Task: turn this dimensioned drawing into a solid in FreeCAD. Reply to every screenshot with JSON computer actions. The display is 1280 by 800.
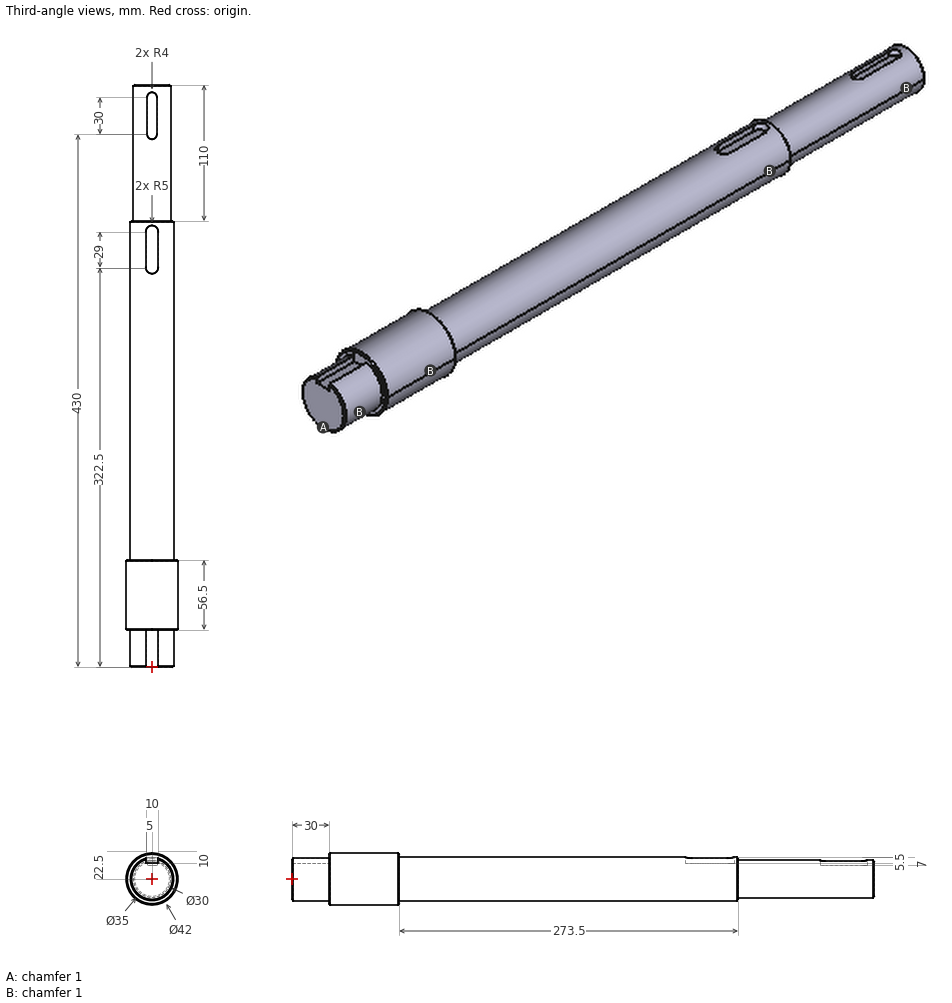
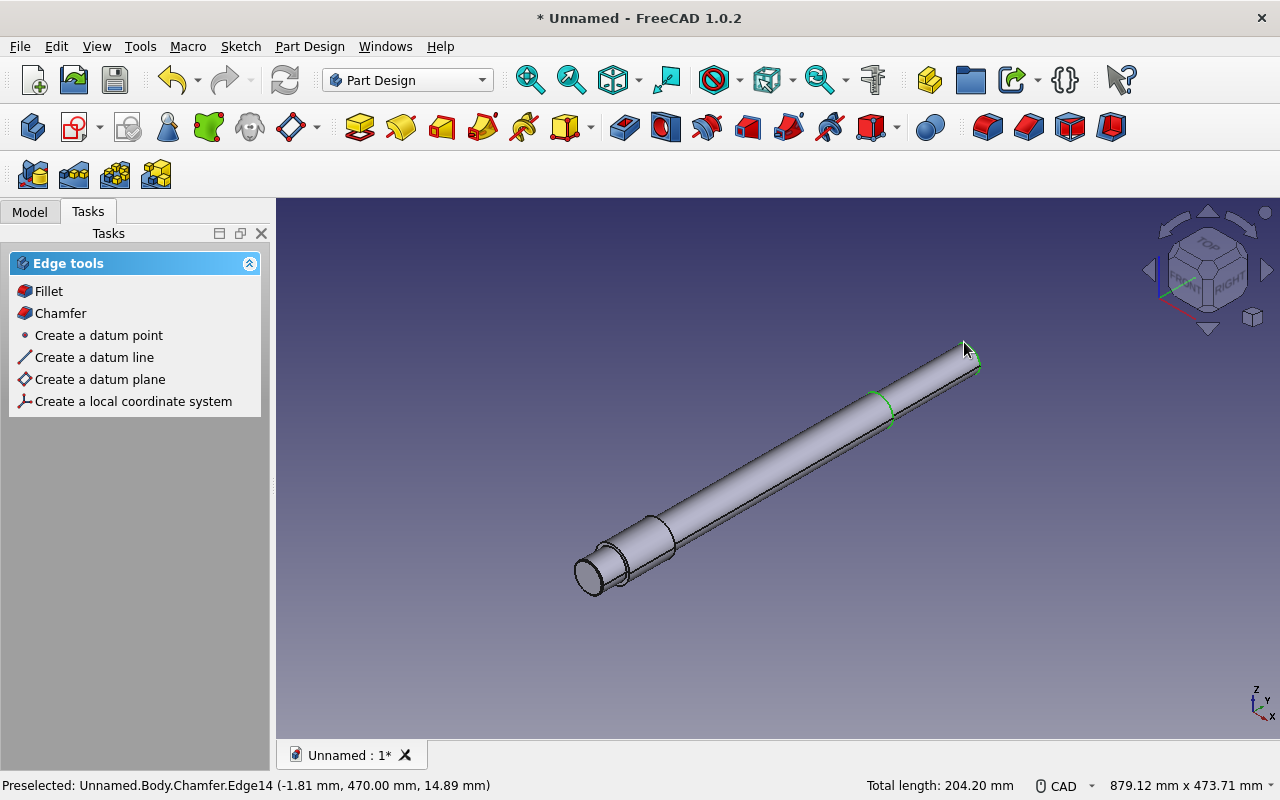
{"action": "left_click", "coordinate": [607, 541], "text": "ctrl"}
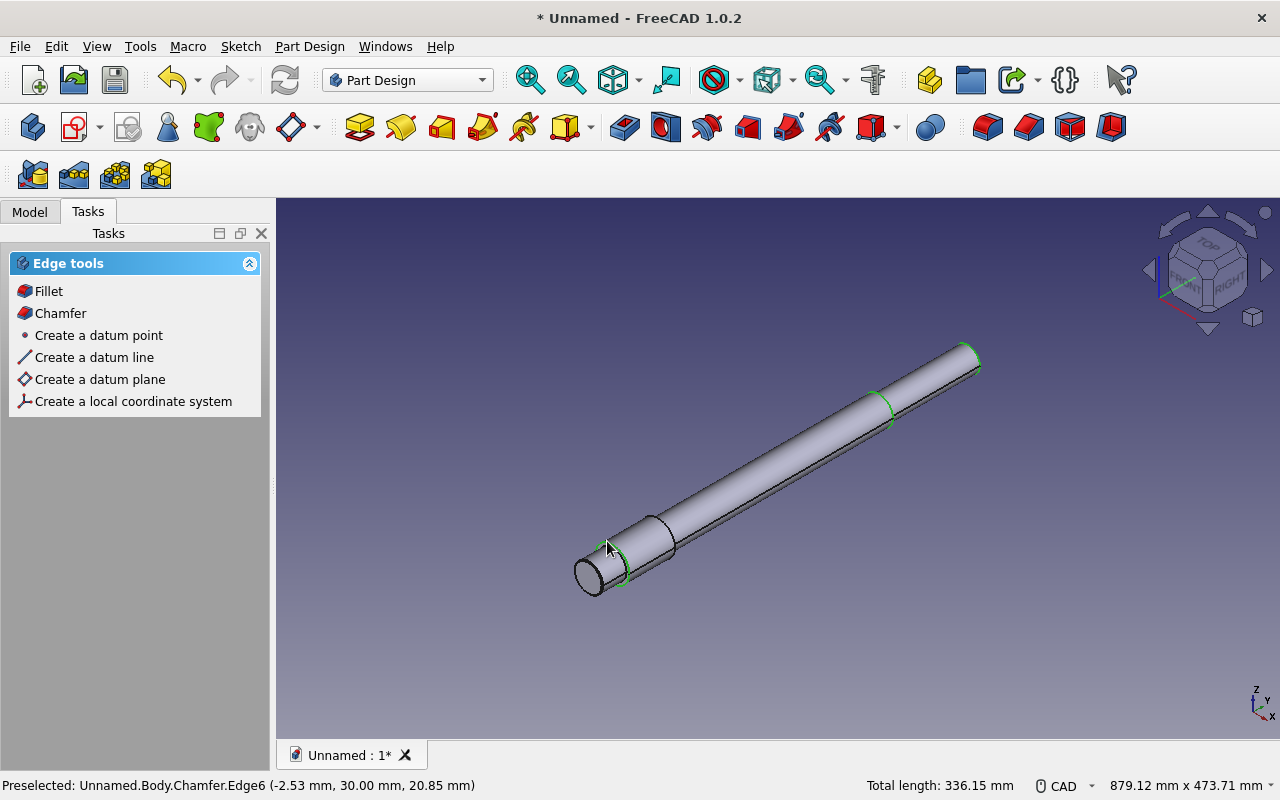
{"action": "left_click", "coordinate": [653, 515], "text": "ctrl"}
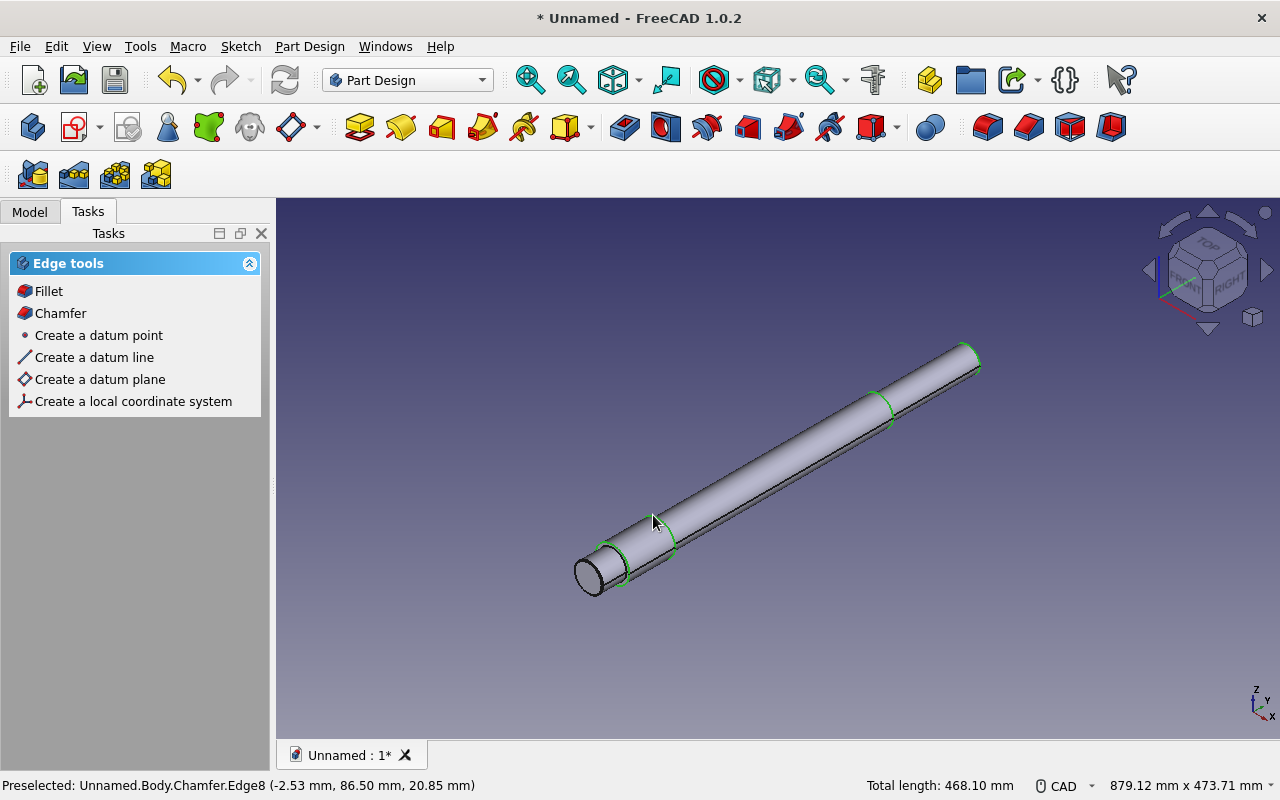
{"action": "left_click", "coordinate": [1029, 128]}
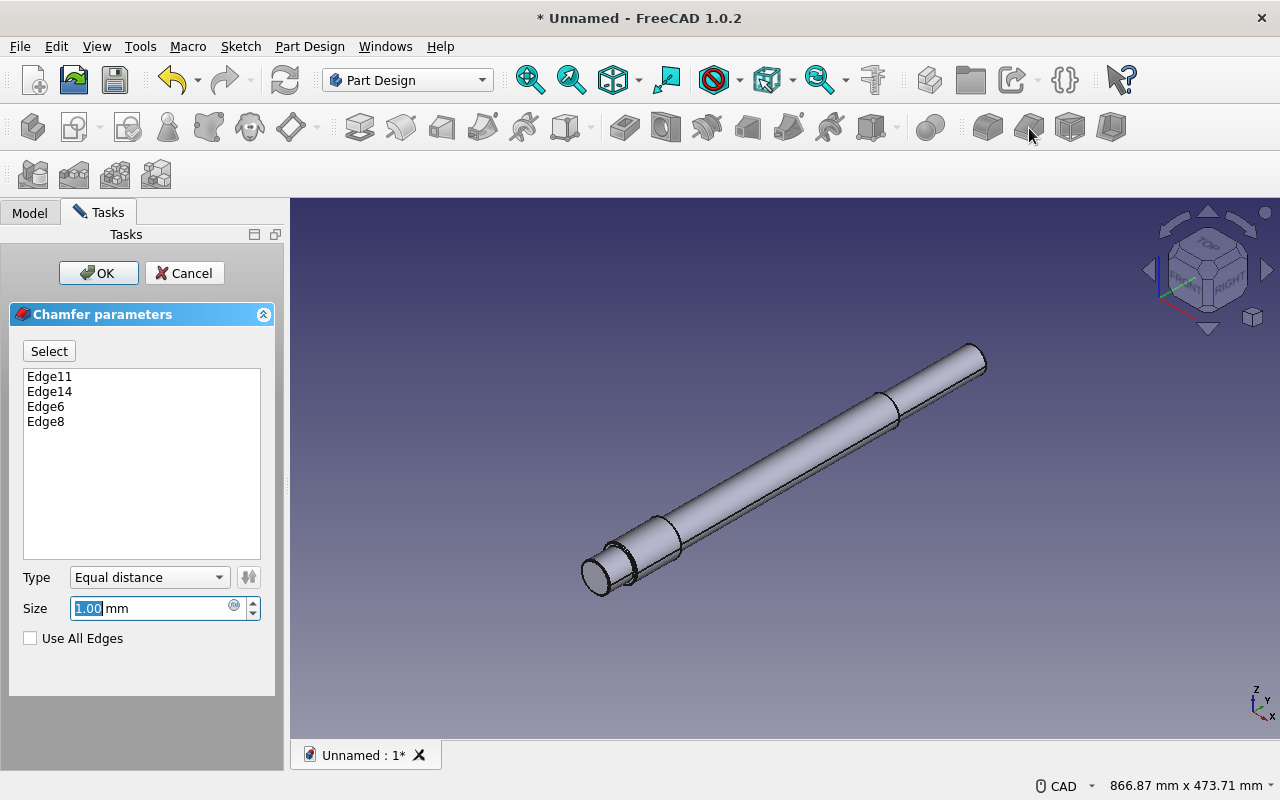
{"action": "type", "text": "1"}
{"action": "key", "text": "Tab"}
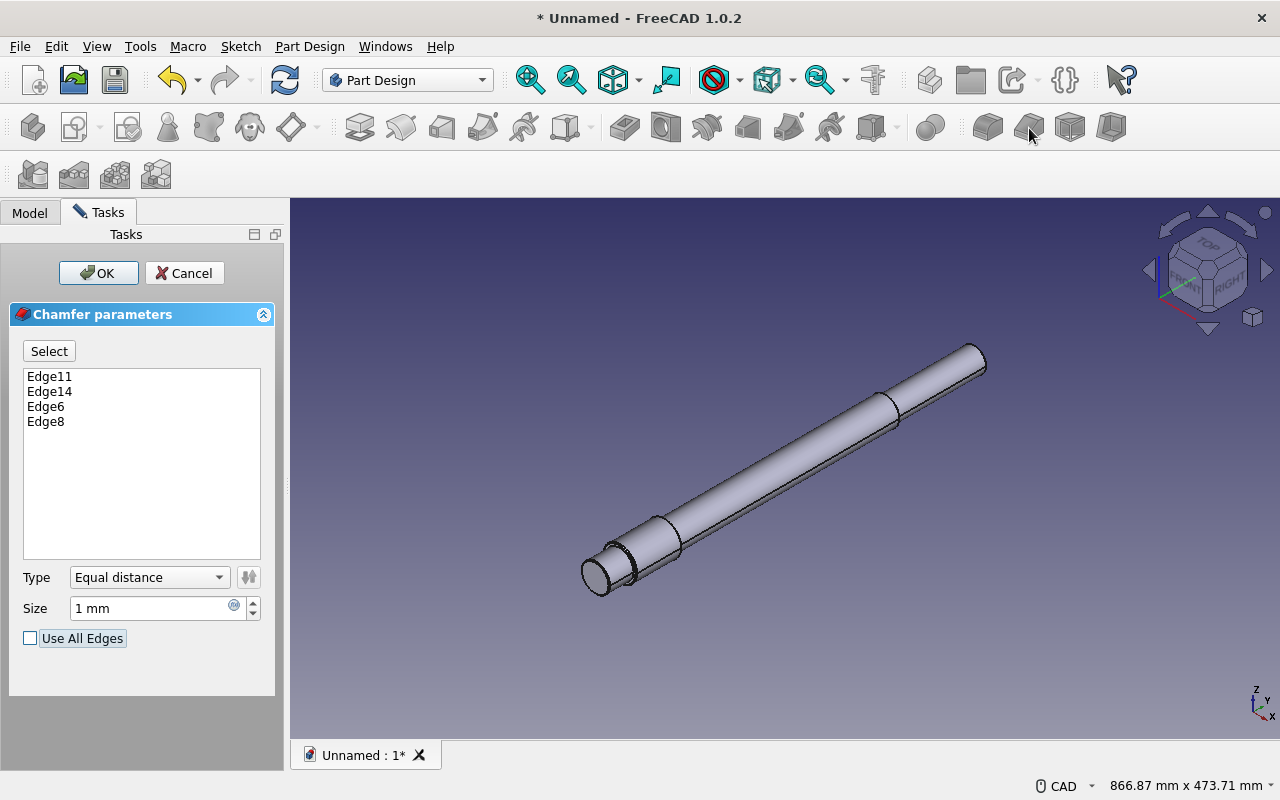
{"action": "left_click", "coordinate": [99, 273]}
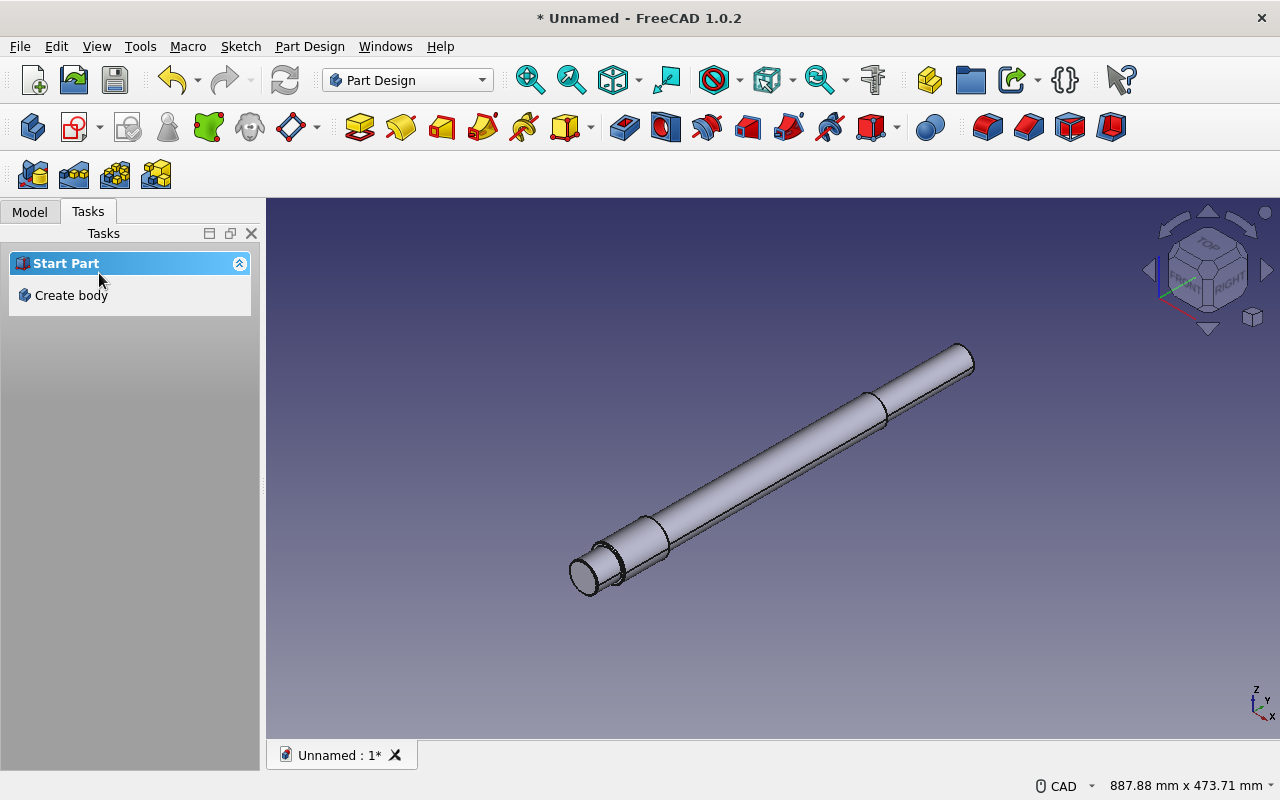
{"action": "left_click", "coordinate": [583, 577]}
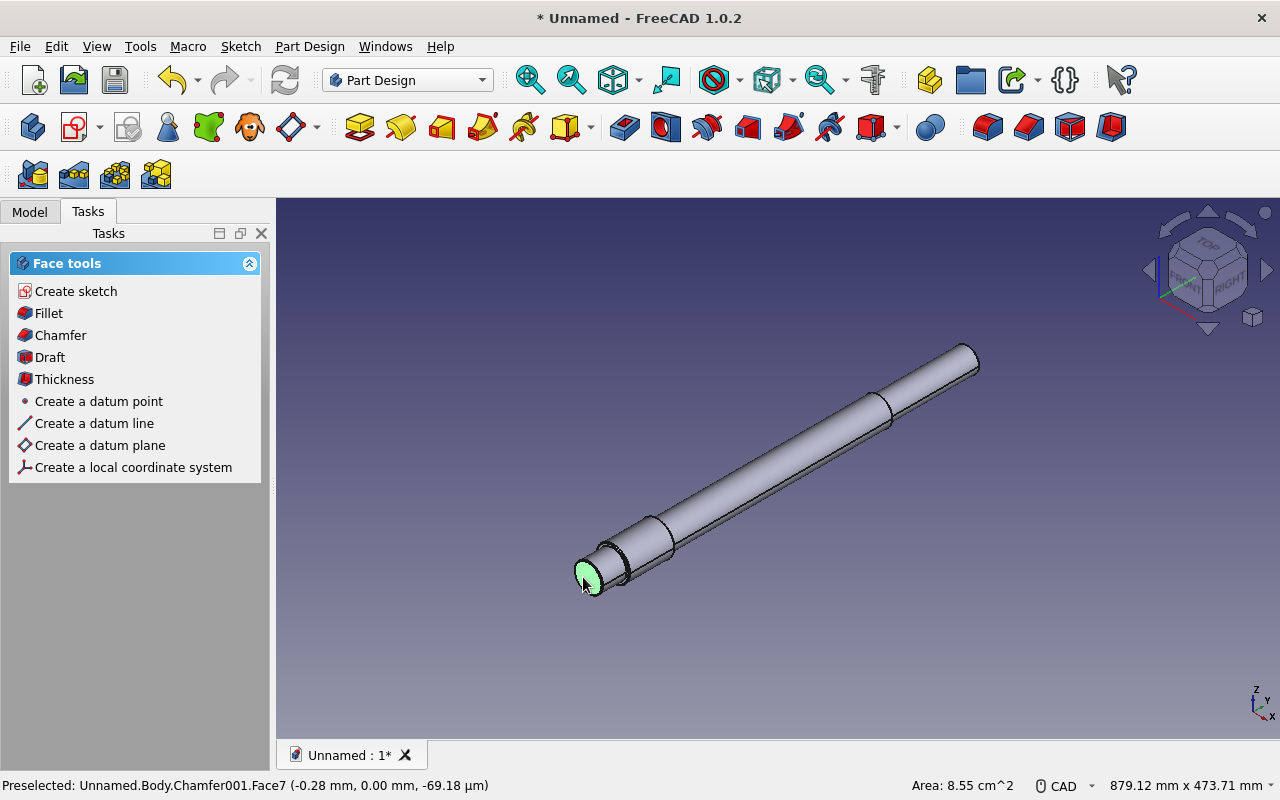
{"action": "left_click", "coordinate": [74, 128]}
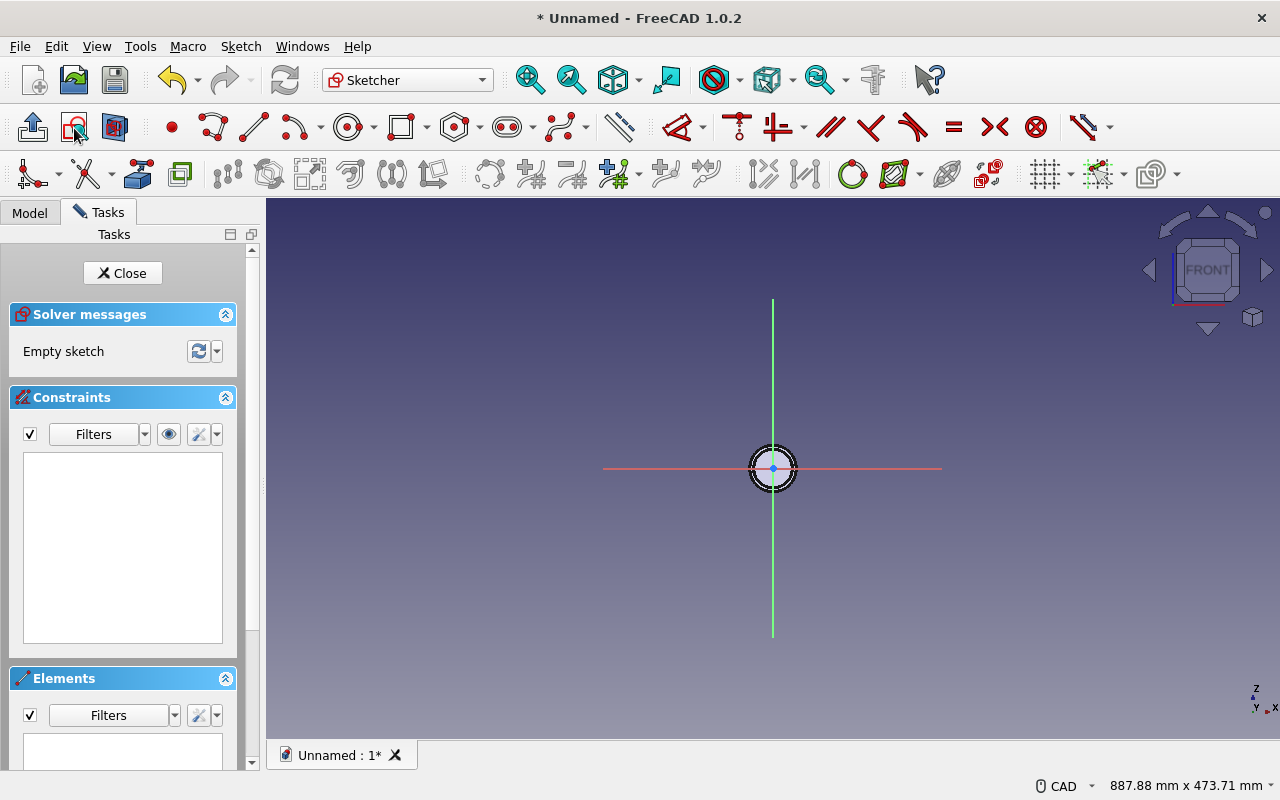
{"action": "scroll", "coordinate": [778, 455], "scroll_direction": "up", "scroll_amount": 13}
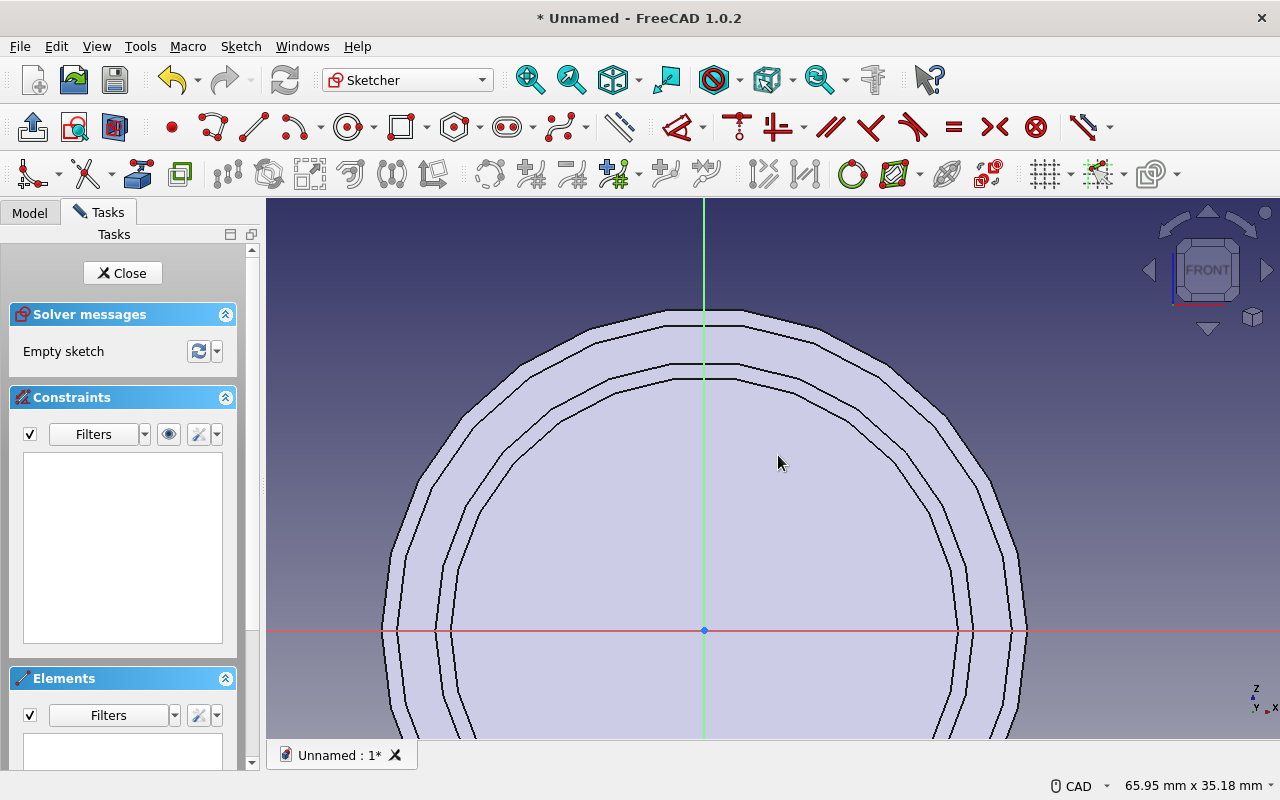
{"action": "key", "text": "g r"}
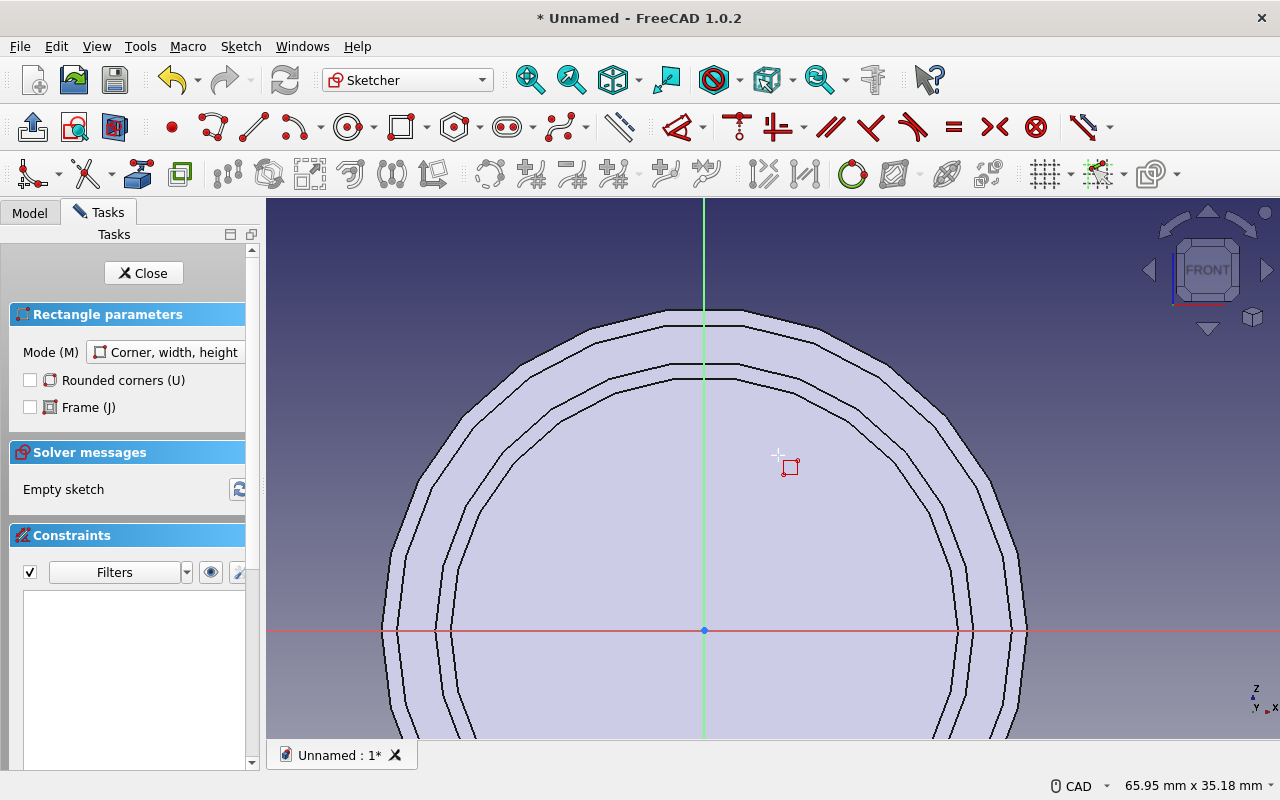
{"action": "left_click", "coordinate": [628, 285]}
{"action": "mouse_move", "coordinate": [781, 439]}